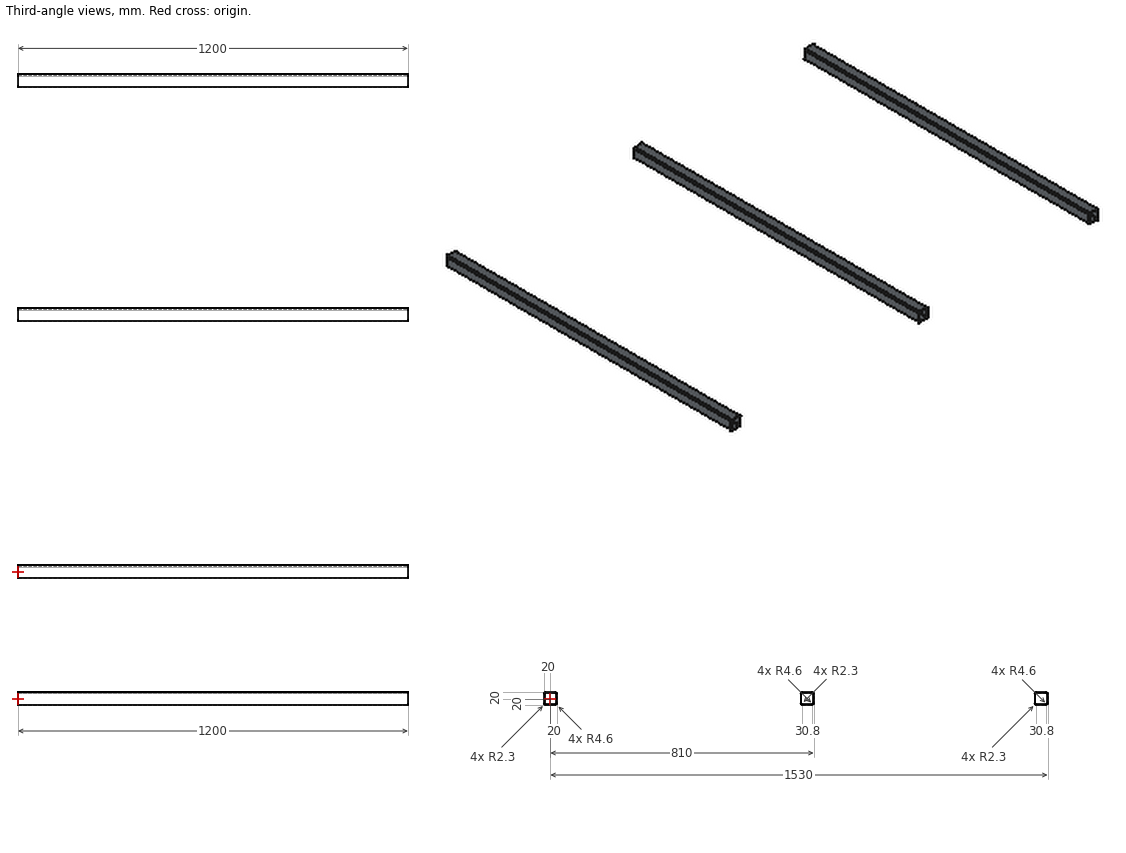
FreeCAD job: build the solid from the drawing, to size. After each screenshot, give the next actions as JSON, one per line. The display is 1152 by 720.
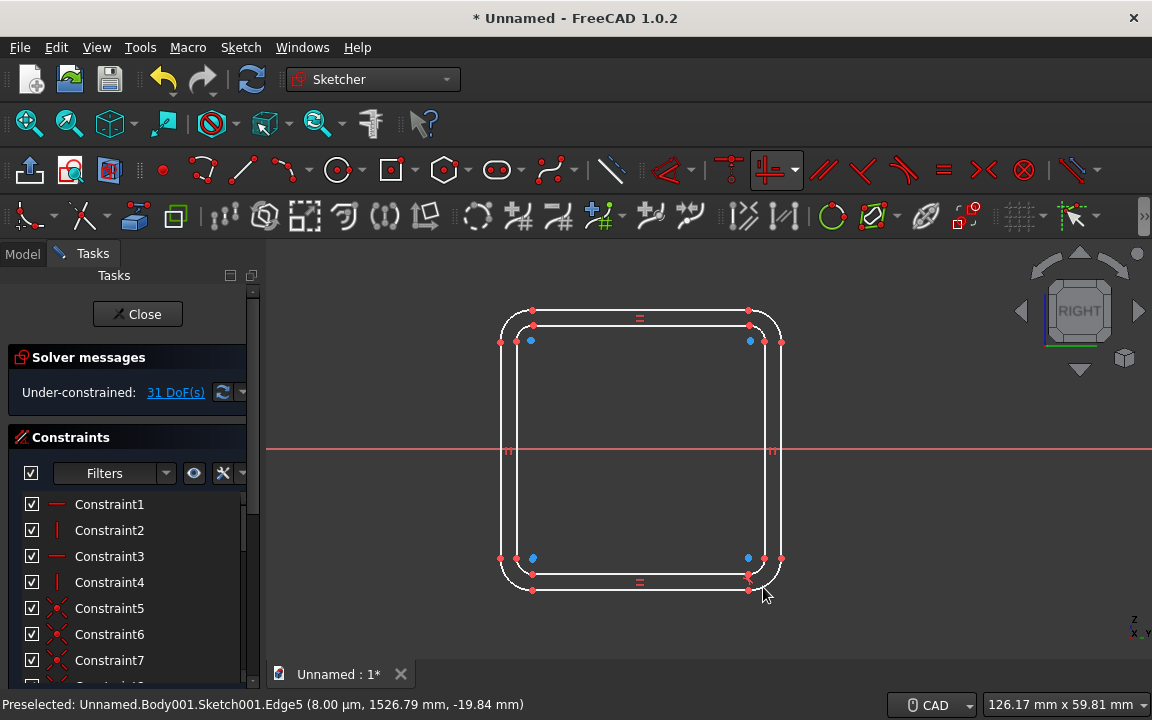
{"action": "left_click", "coordinate": [598, 590]}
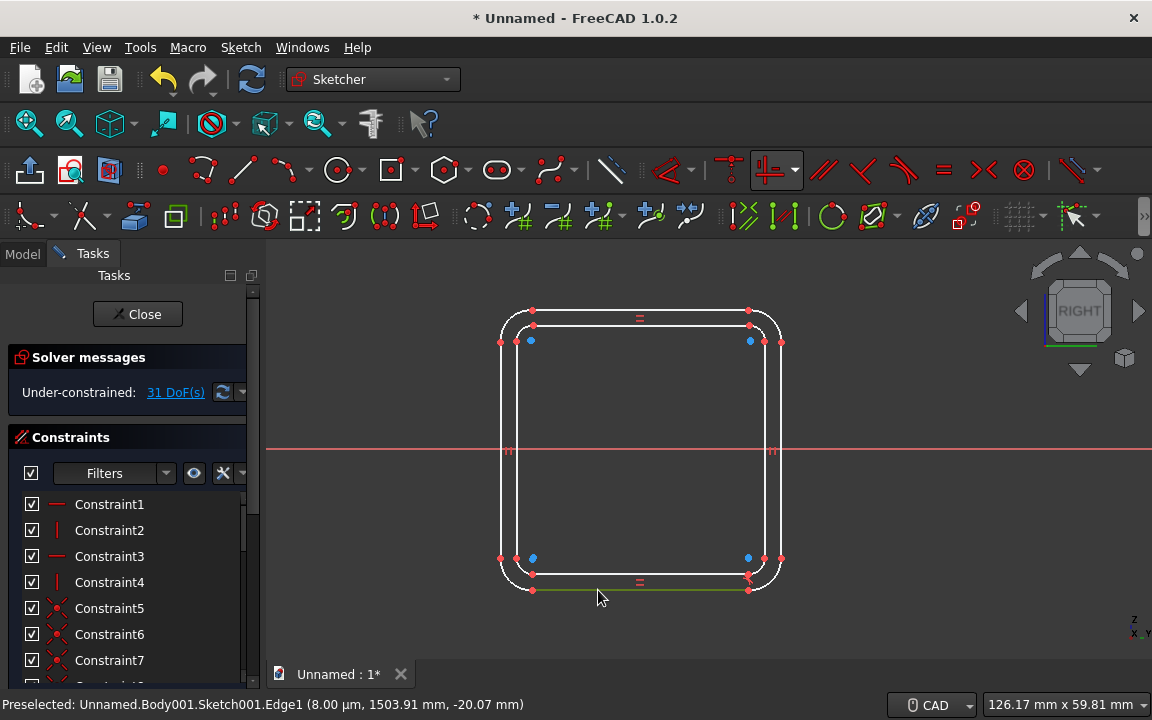
{"action": "left_click", "coordinate": [504, 573]}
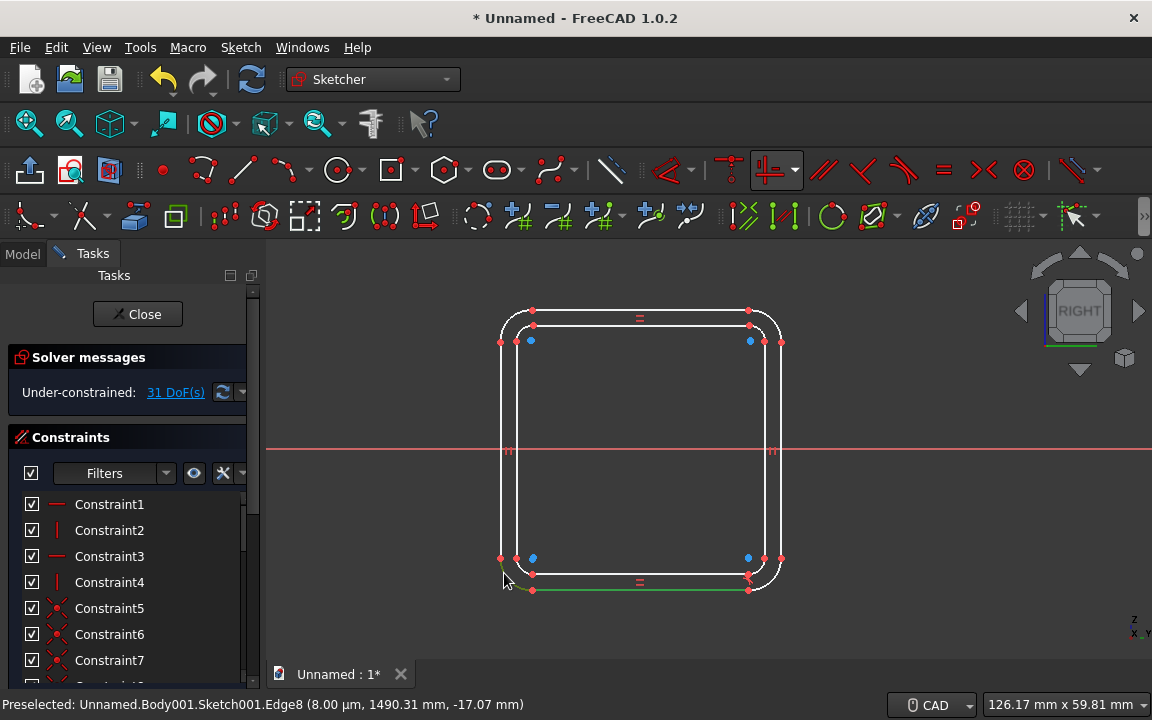
{"action": "key", "text": "t"}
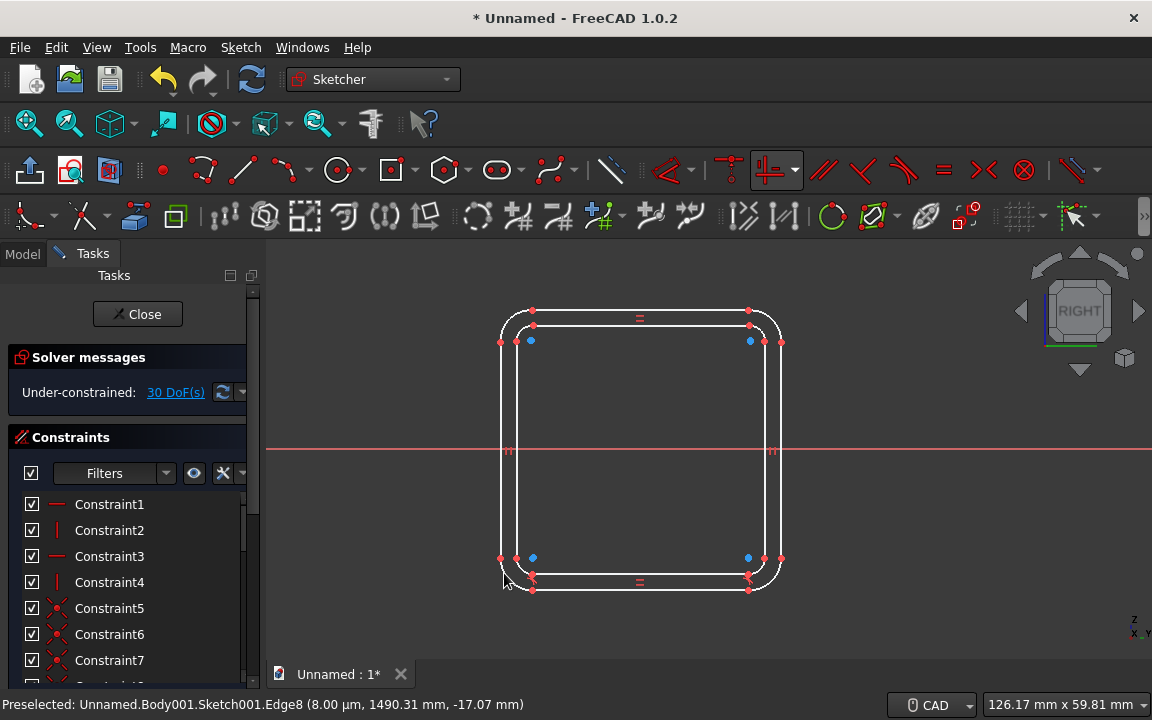
{"action": "left_click", "coordinate": [781, 494]}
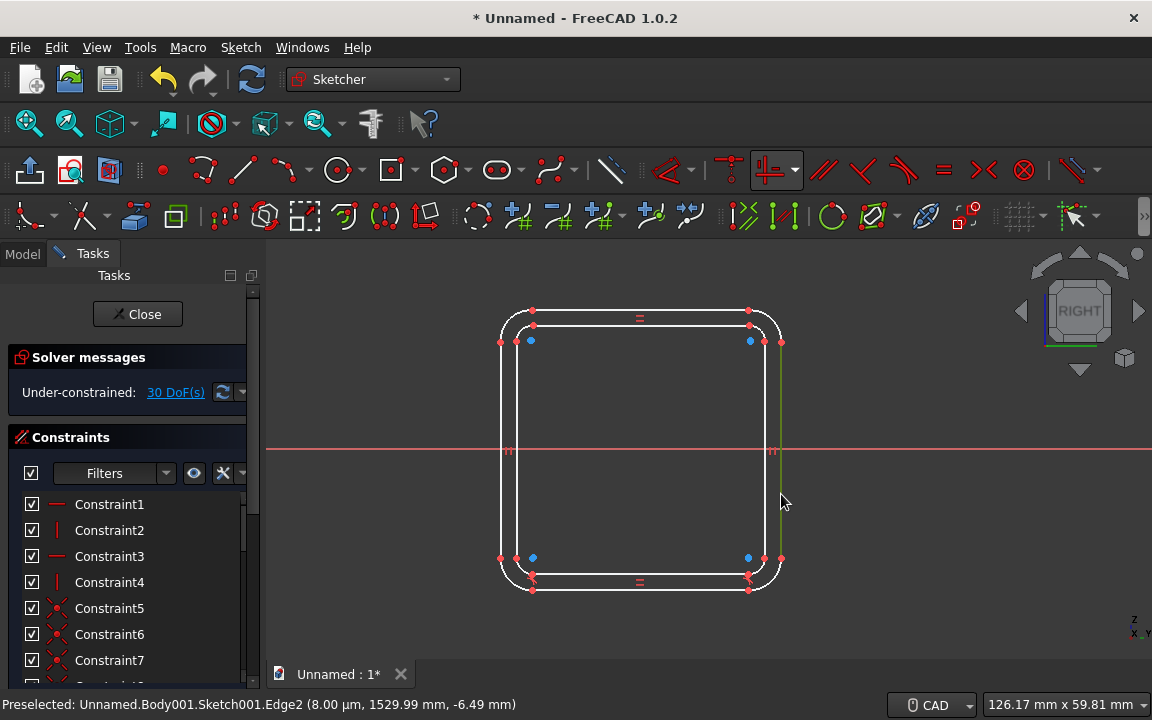
{"action": "left_click", "coordinate": [763, 587]}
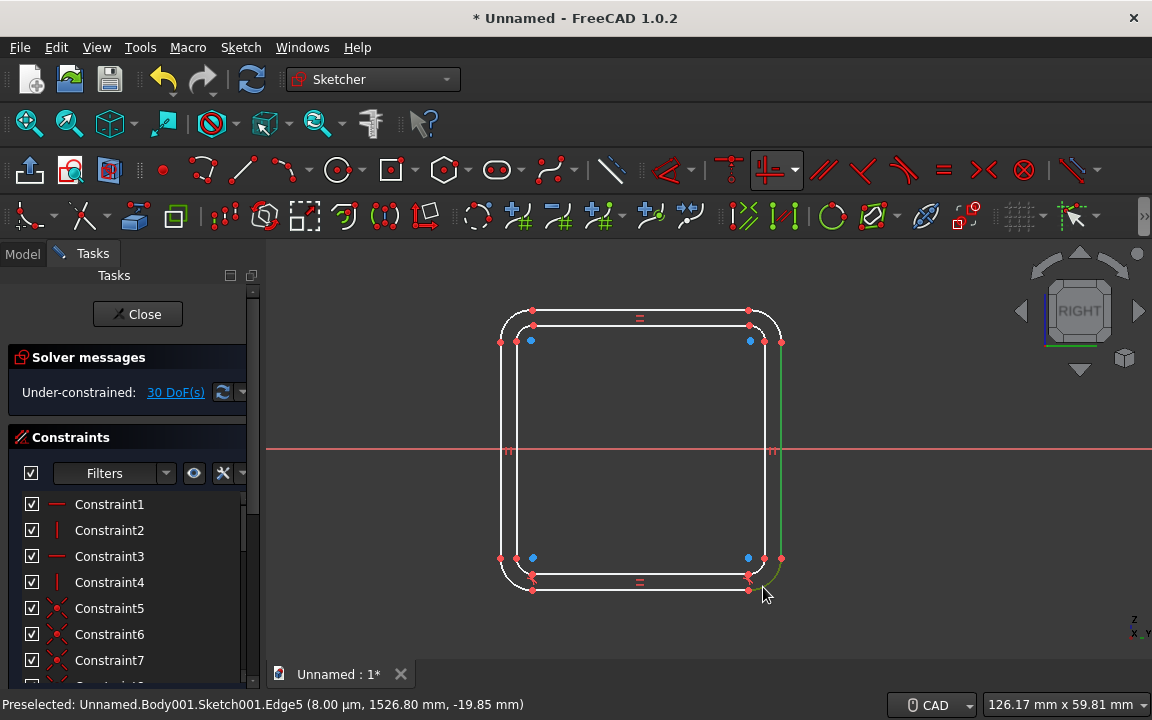
{"action": "left_click", "coordinate": [904, 170]}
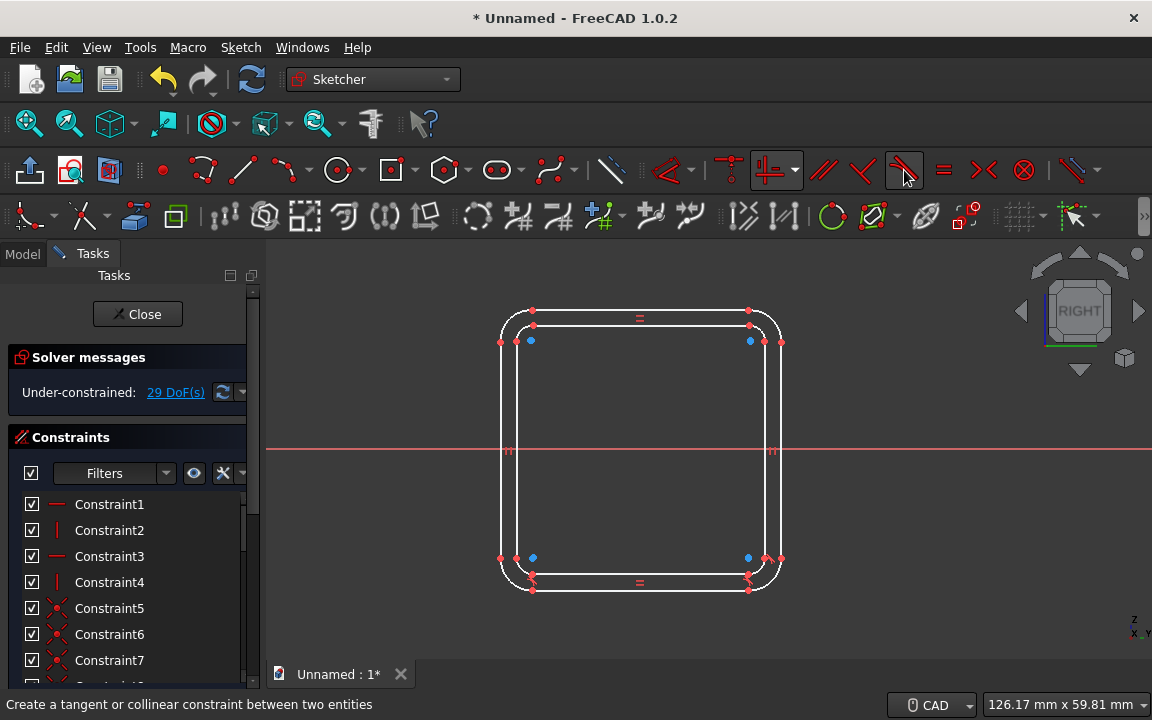
{"action": "left_click", "coordinate": [781, 494]}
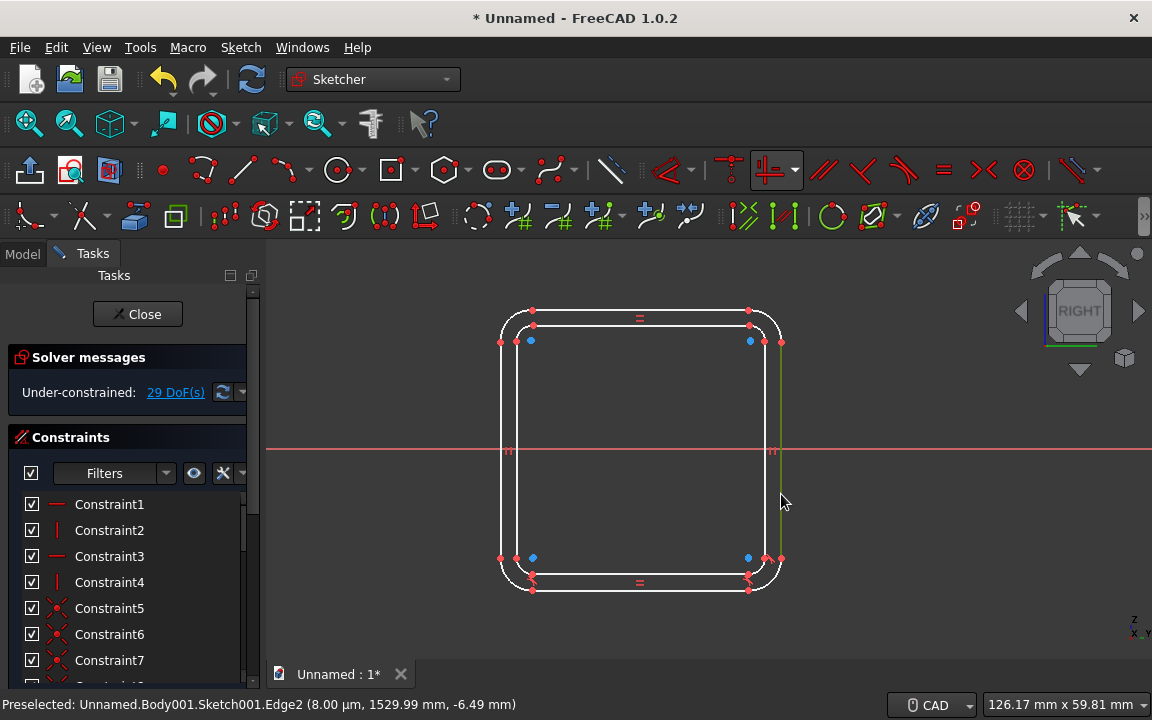
{"action": "left_click", "coordinate": [778, 328]}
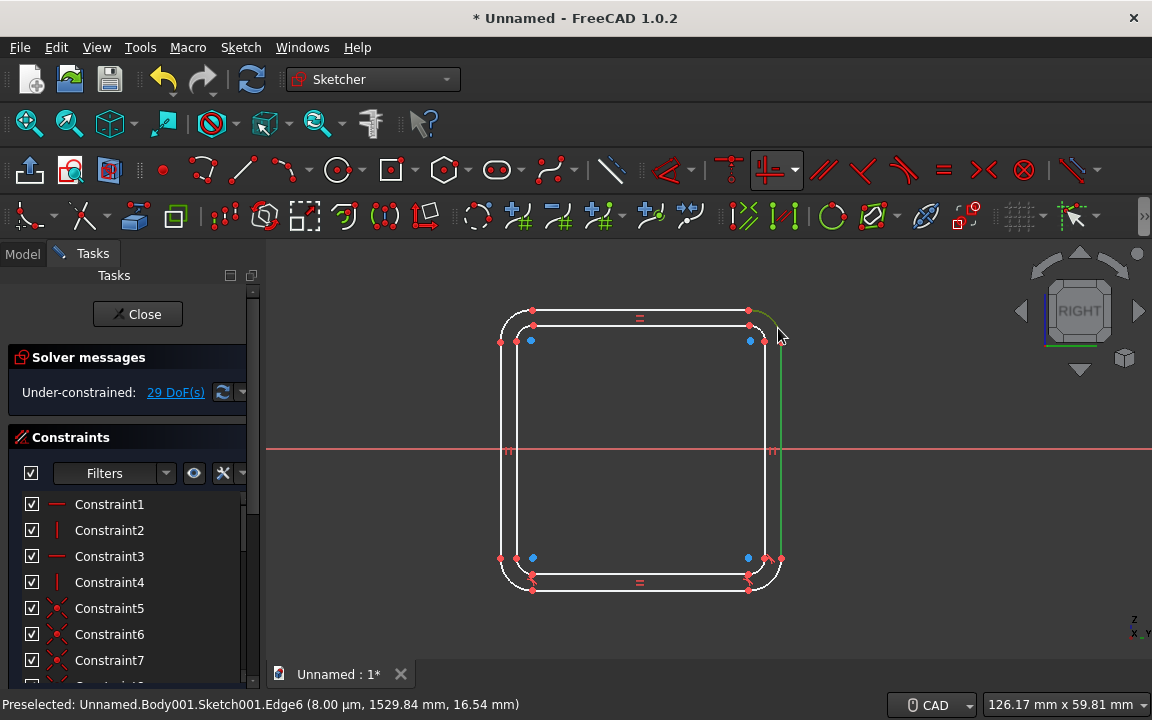
{"action": "left_click", "coordinate": [904, 170]}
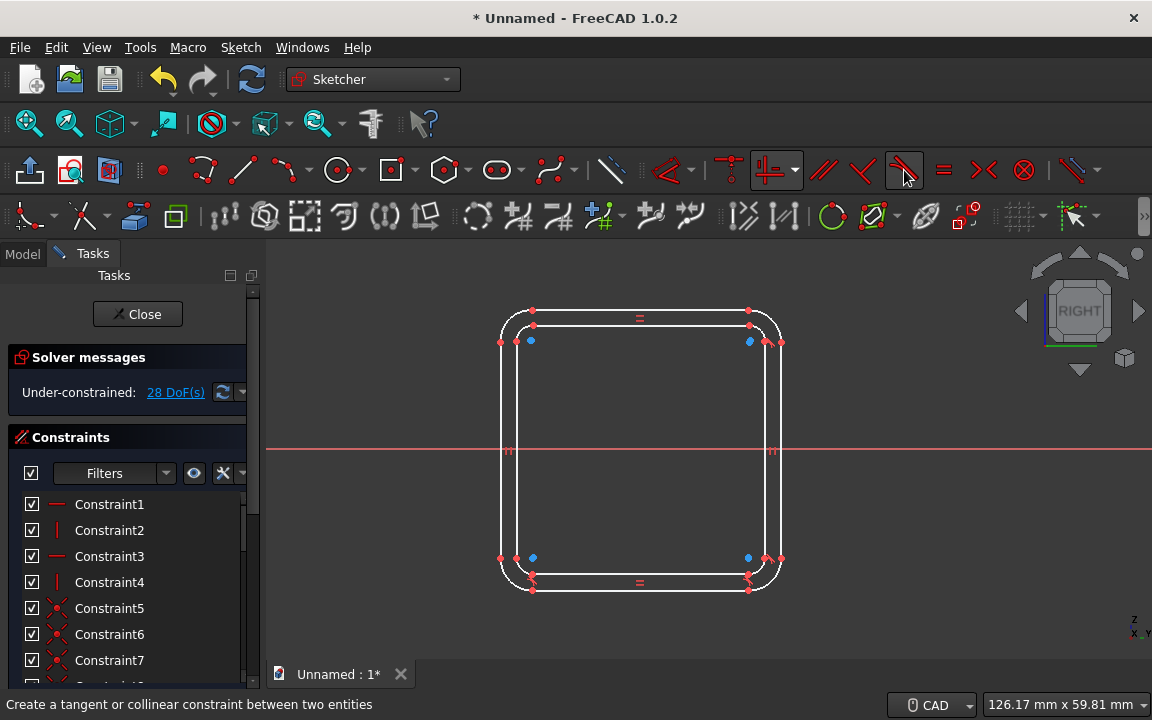
{"action": "left_click", "coordinate": [684, 310]}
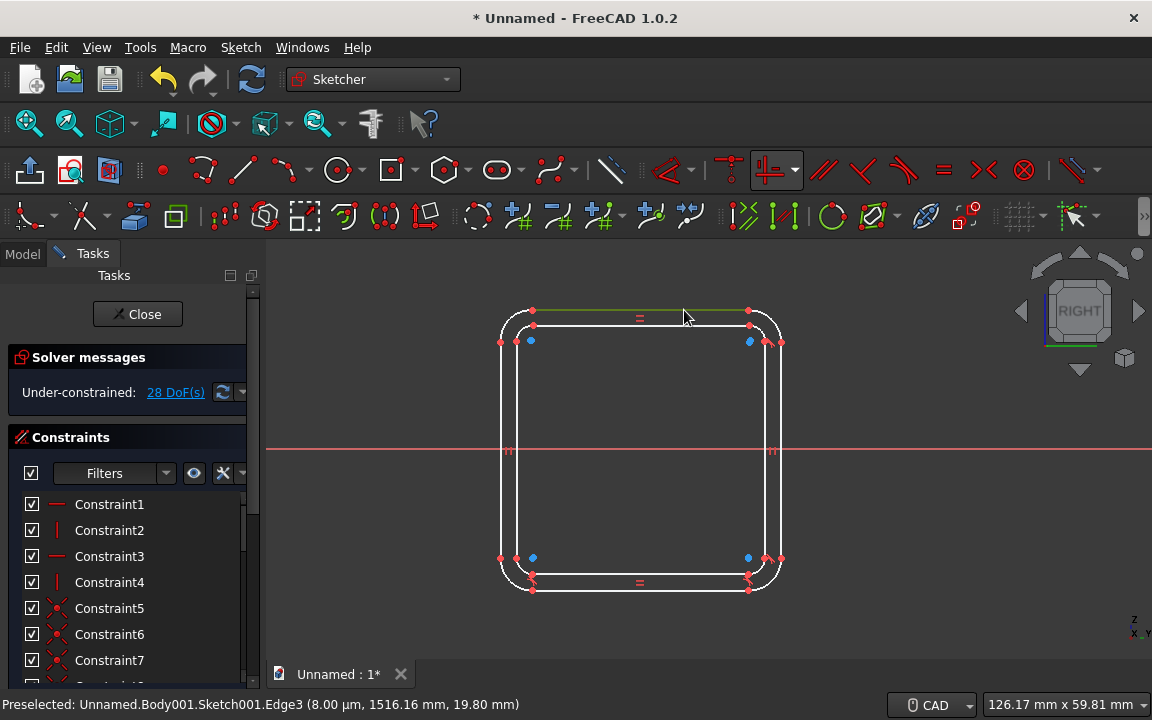
{"action": "left_click", "coordinate": [778, 328]}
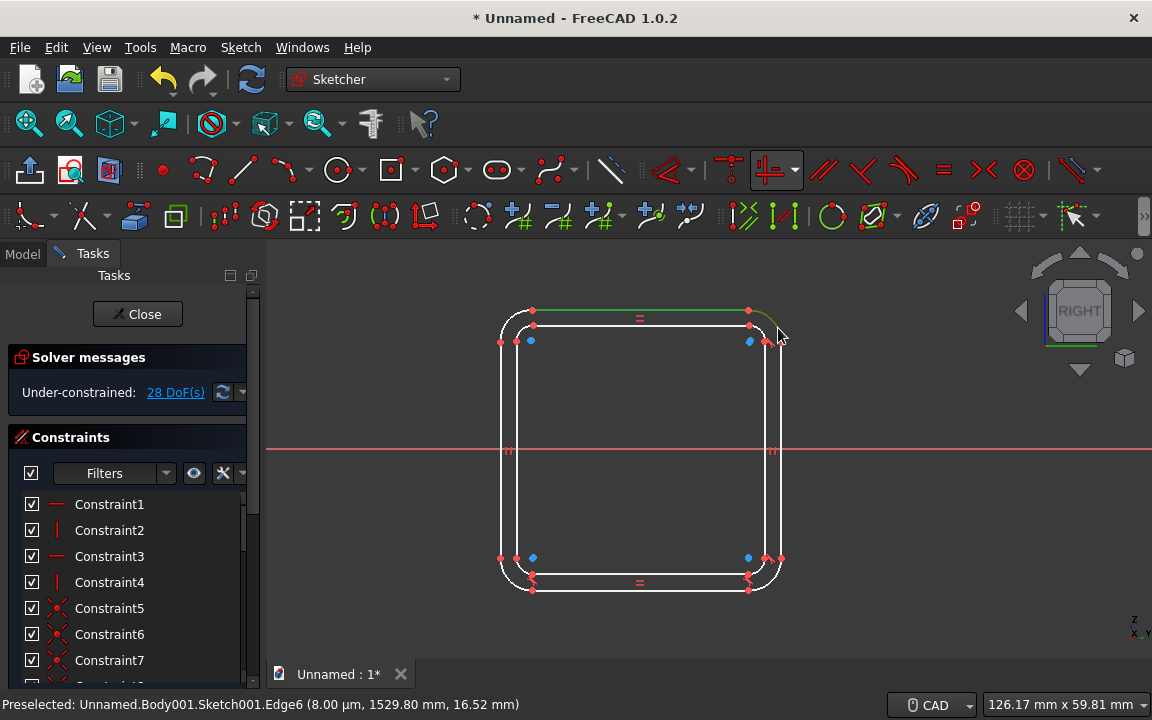
{"action": "left_click", "coordinate": [904, 170]}